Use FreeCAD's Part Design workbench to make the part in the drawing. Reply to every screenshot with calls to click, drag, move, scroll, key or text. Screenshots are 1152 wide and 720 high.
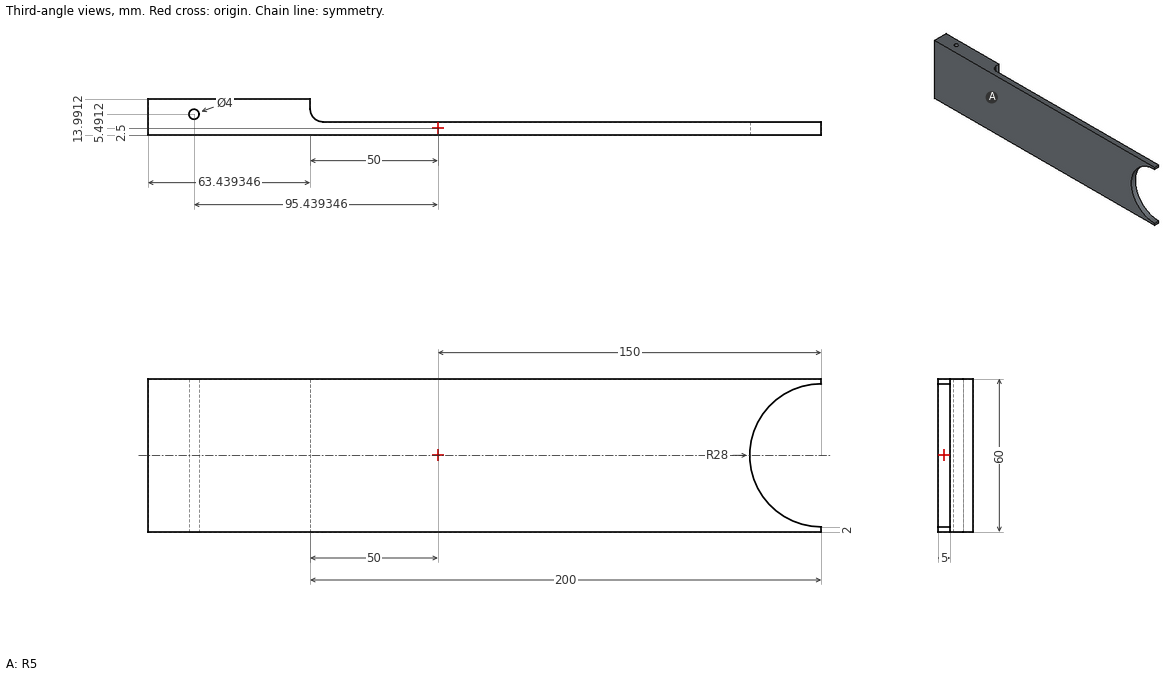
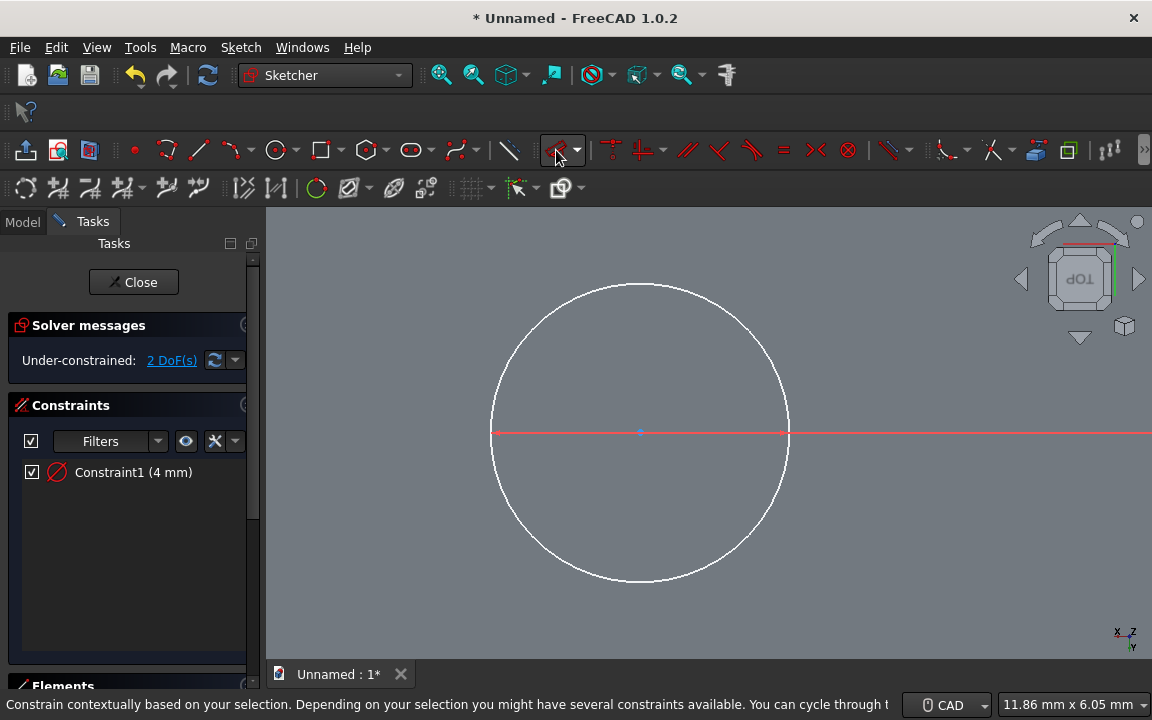
click(640, 433)
click(674, 334)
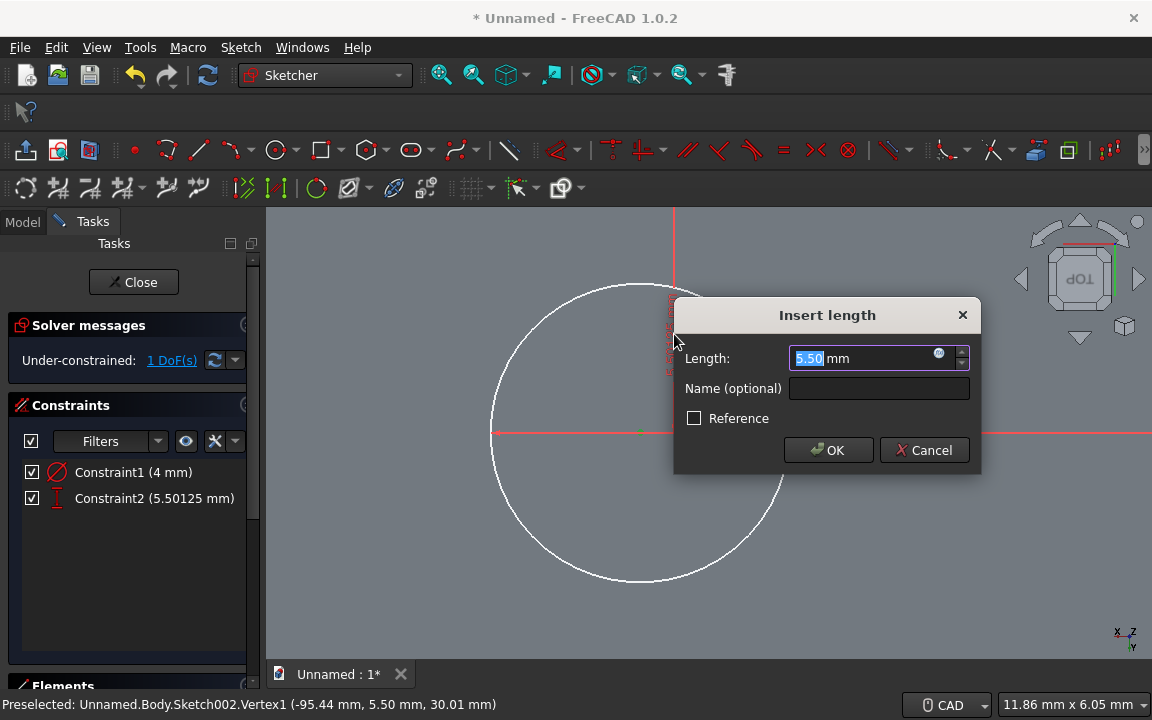
text(5.4912)
key(Return)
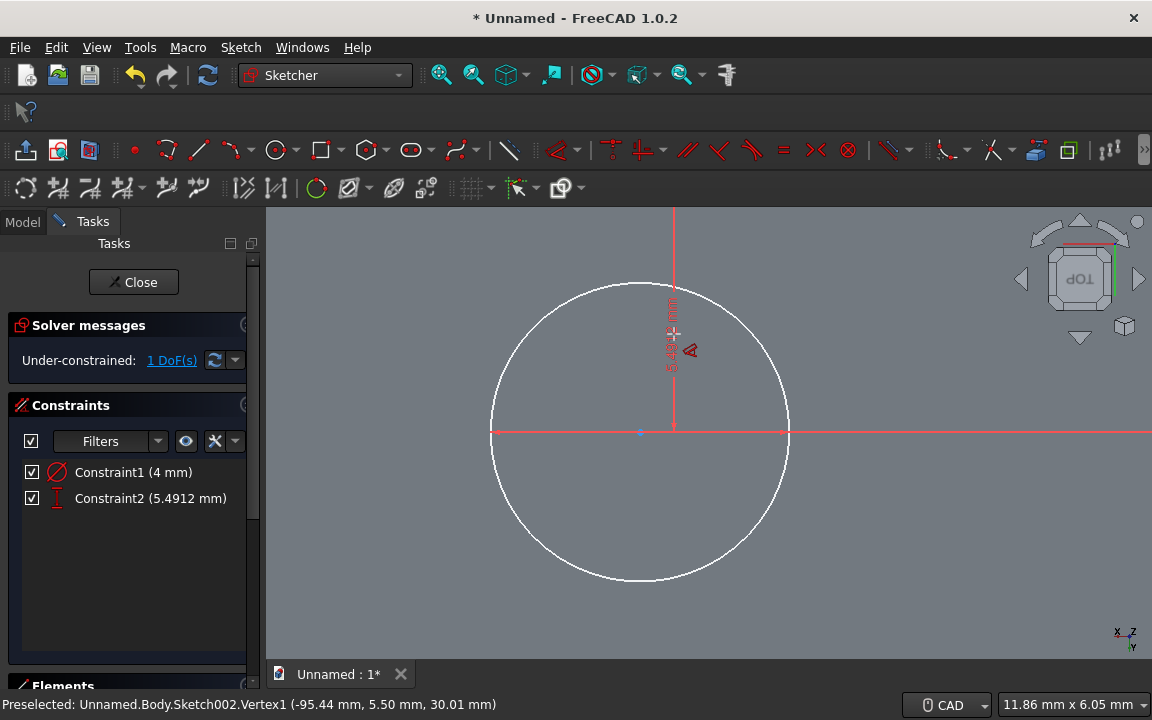
click(640, 432)
click(467, 466)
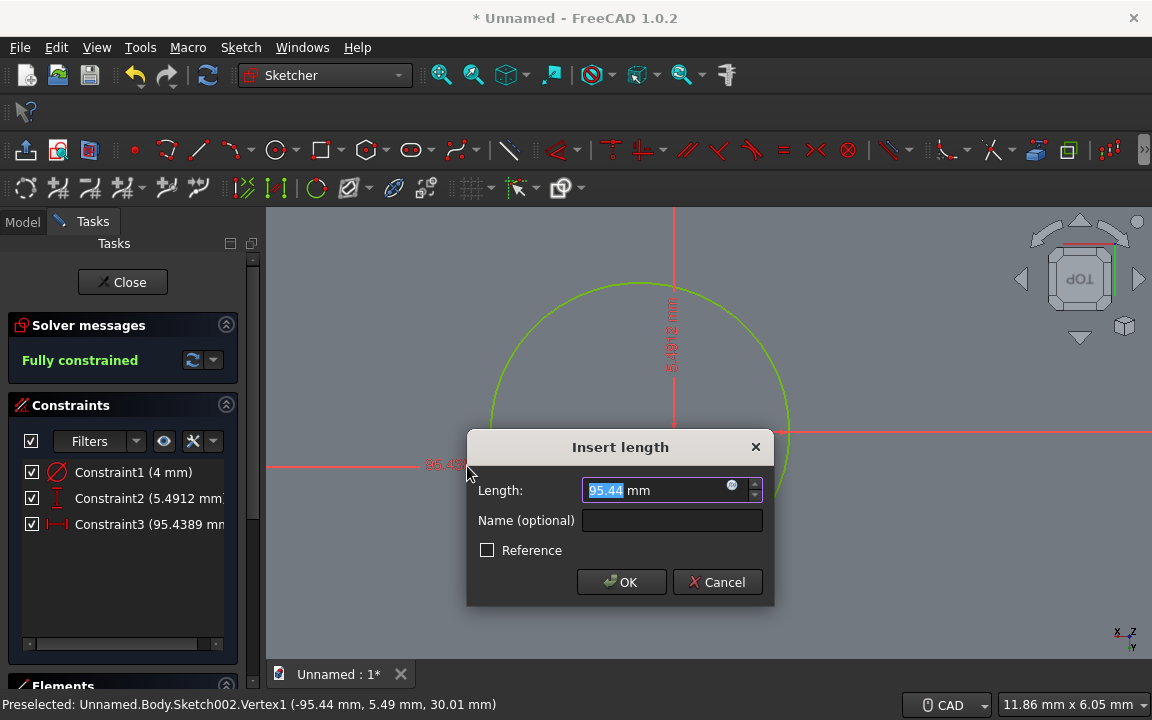
text(95.439346)
key(Return)
key(Escape)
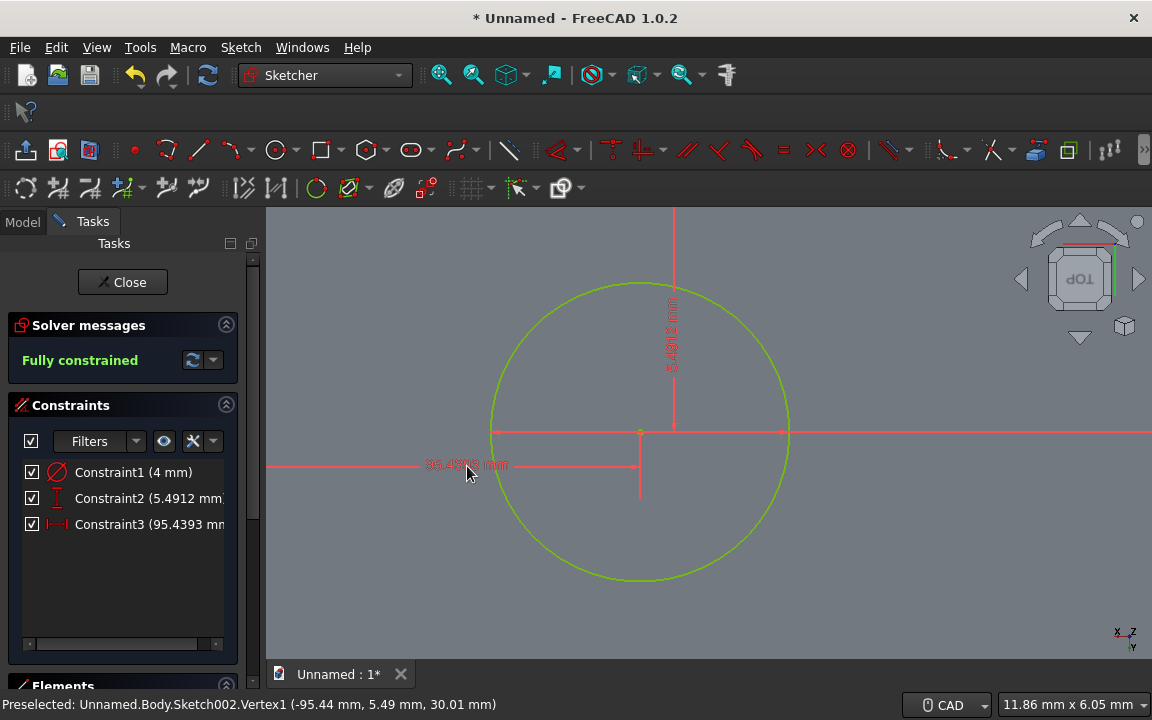
click(123, 282)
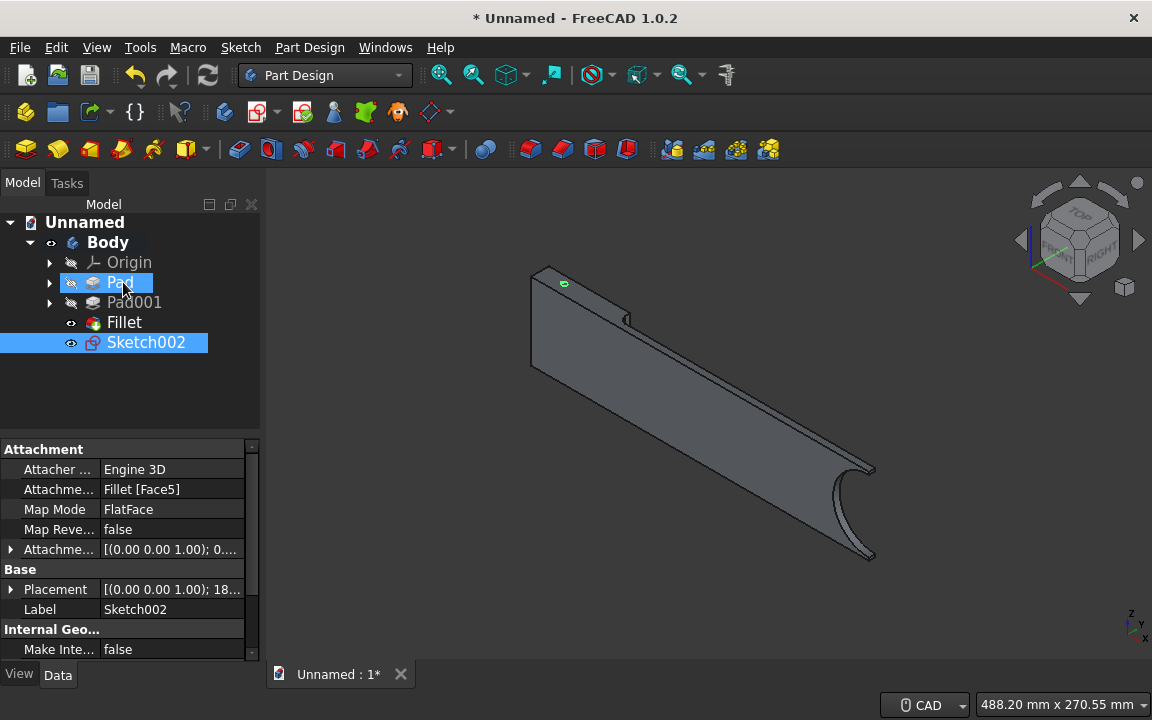
click(240, 150)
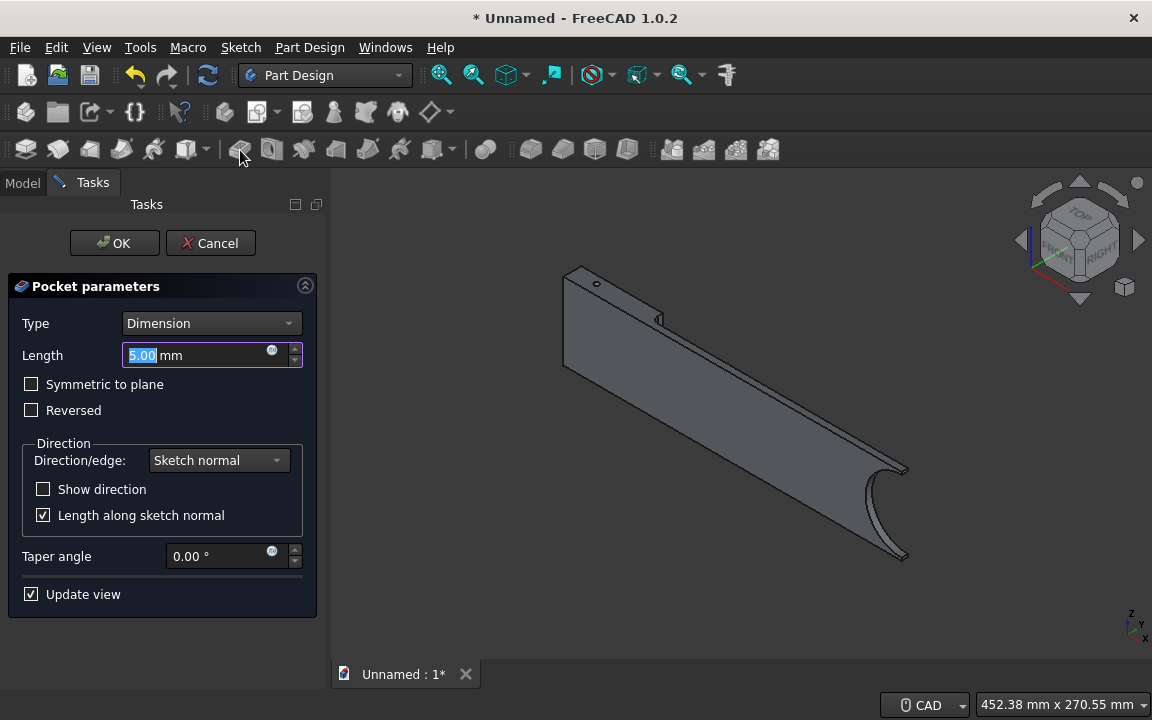
click(212, 324)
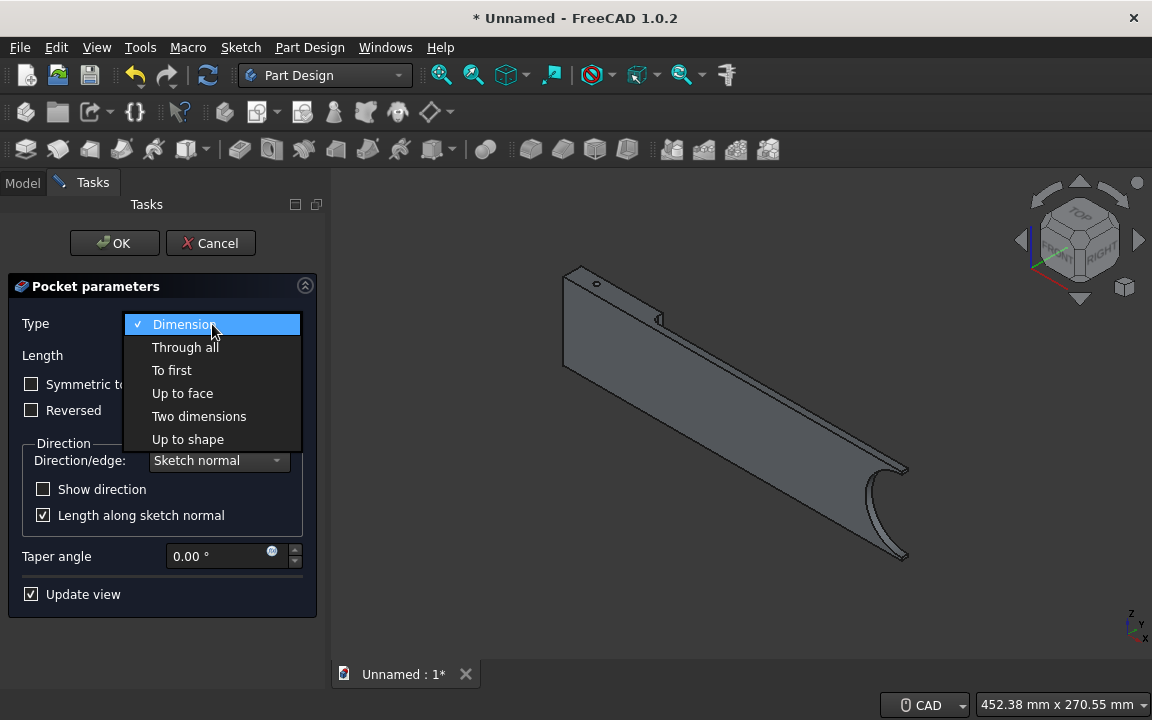
click(212, 348)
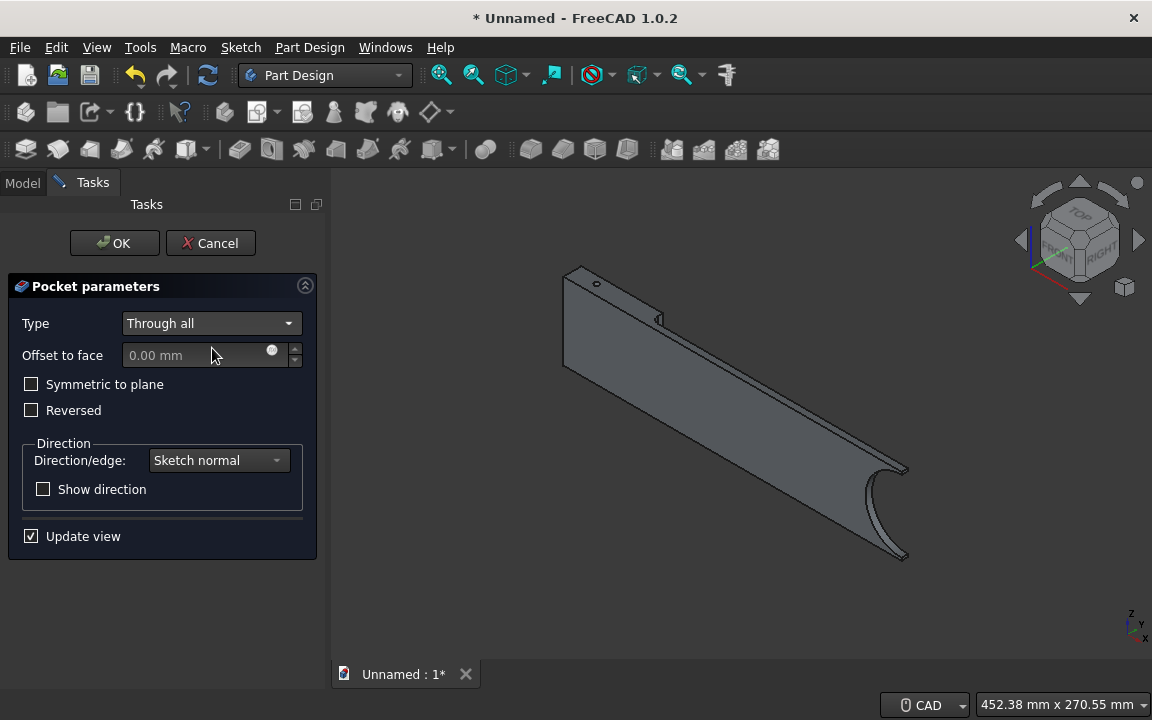
click(115, 243)